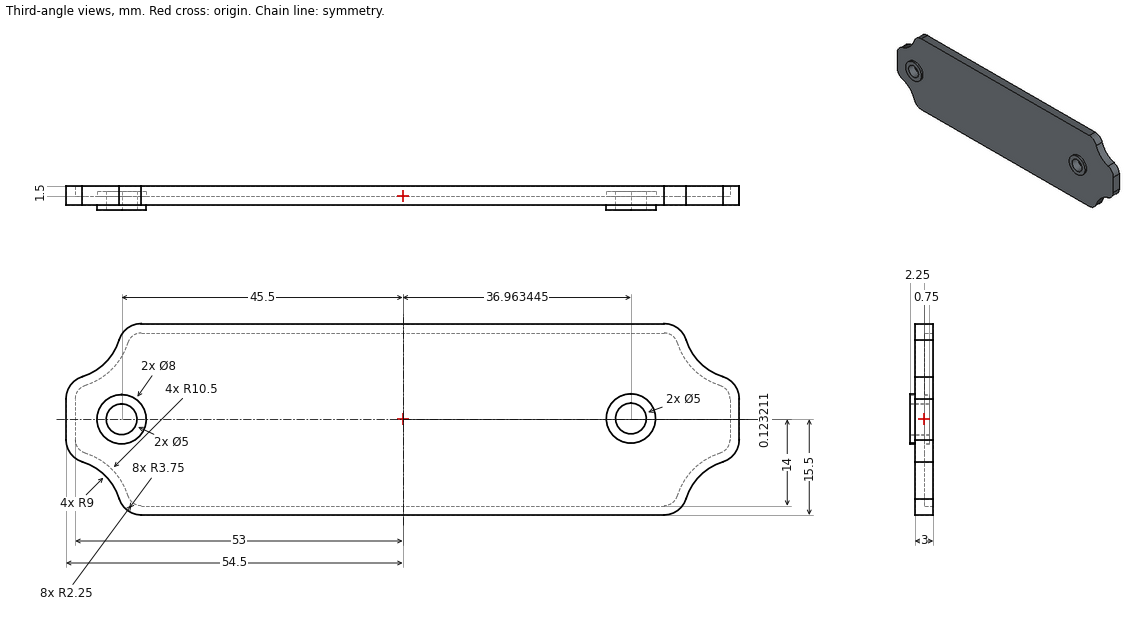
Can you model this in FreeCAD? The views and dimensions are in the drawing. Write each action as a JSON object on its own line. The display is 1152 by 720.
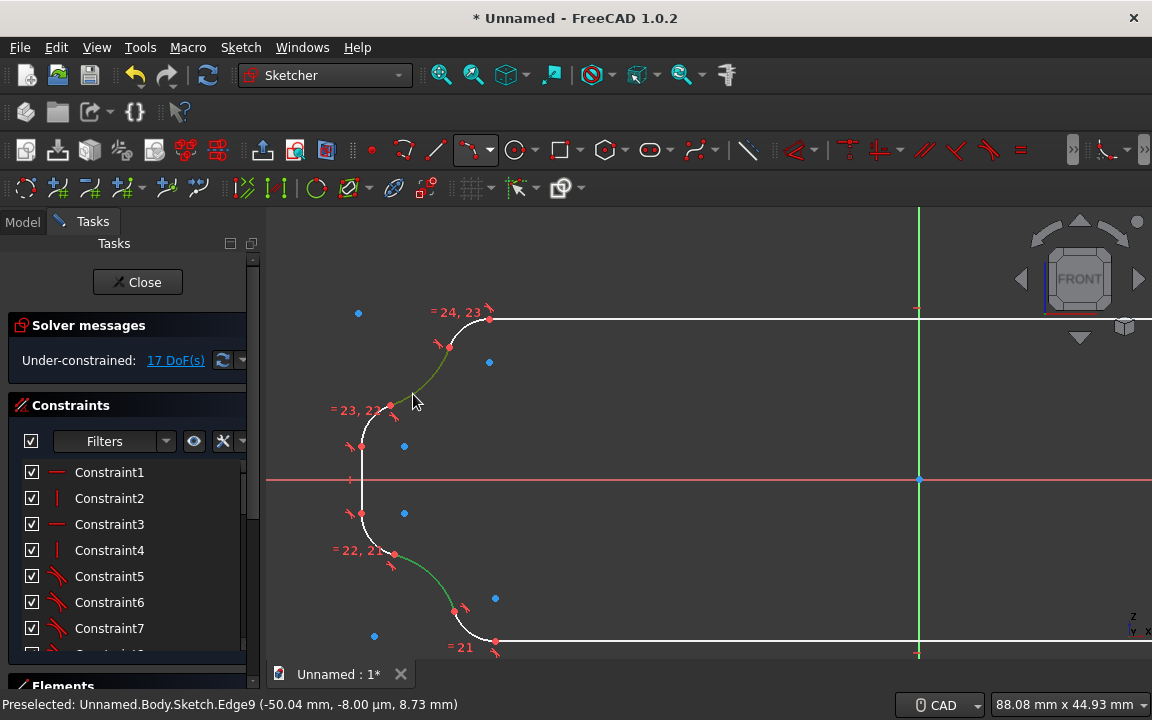
{"action": "scroll", "coordinate": [413, 395], "scroll_direction": "down", "scroll_amount": 4}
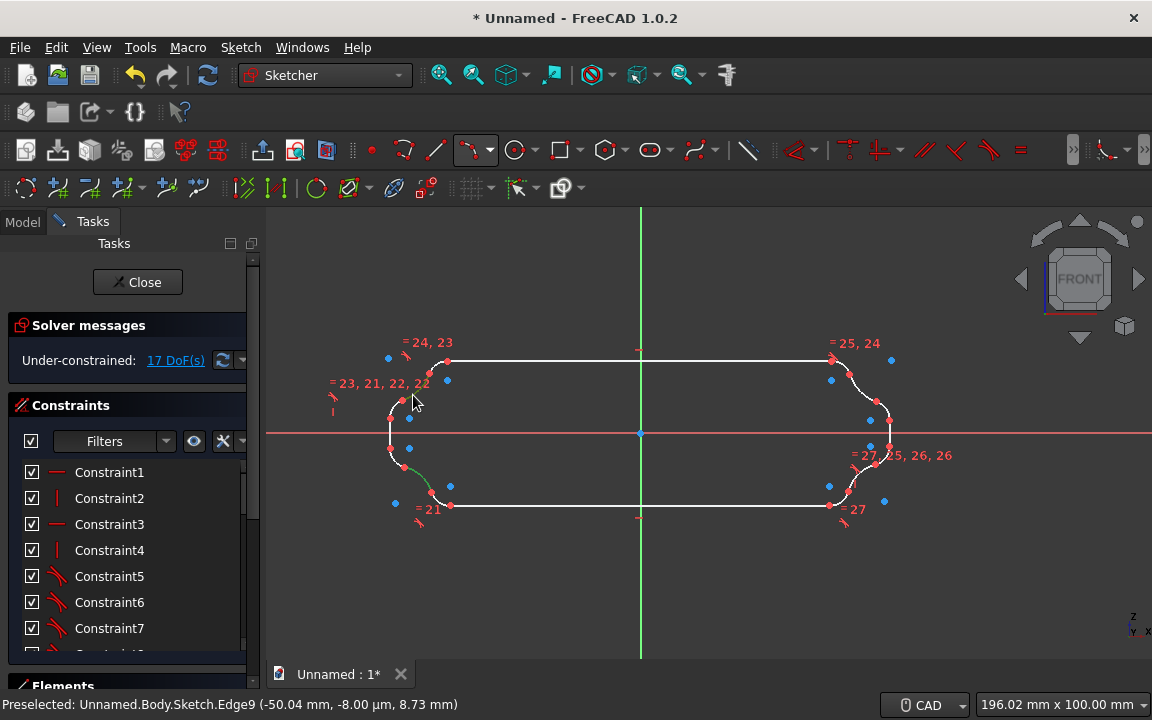
{"action": "left_click", "coordinate": [855, 385]}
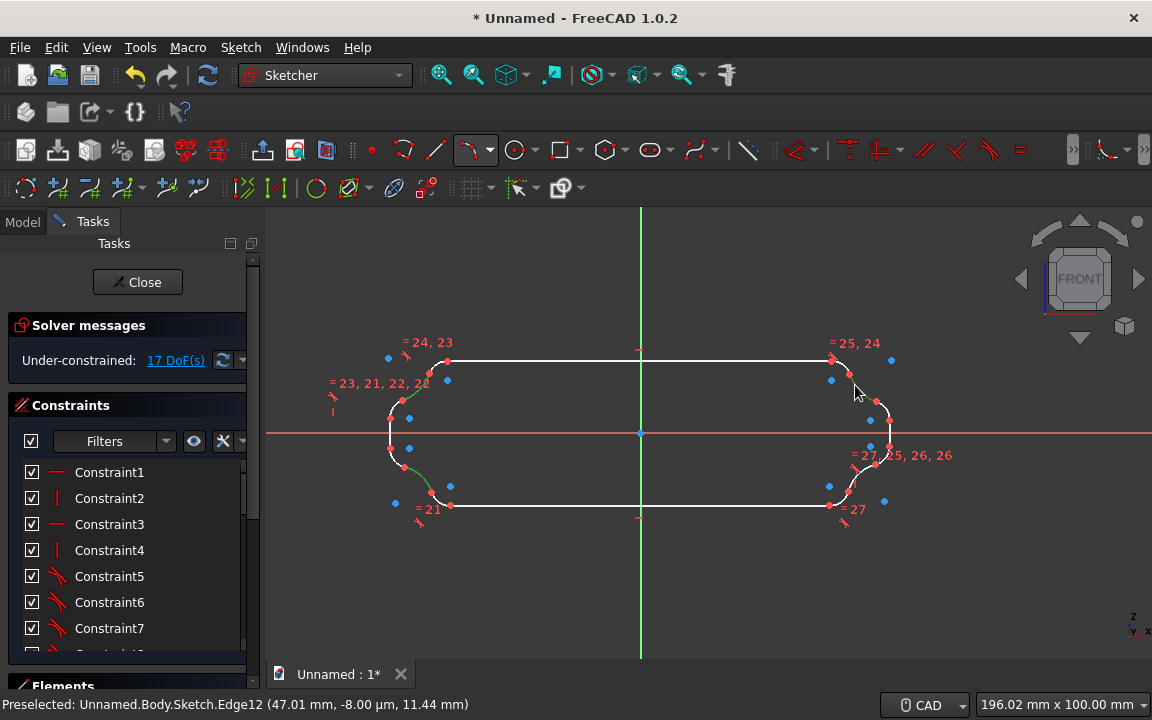
{"action": "scroll", "coordinate": [864, 470], "scroll_direction": "up", "scroll_amount": 4}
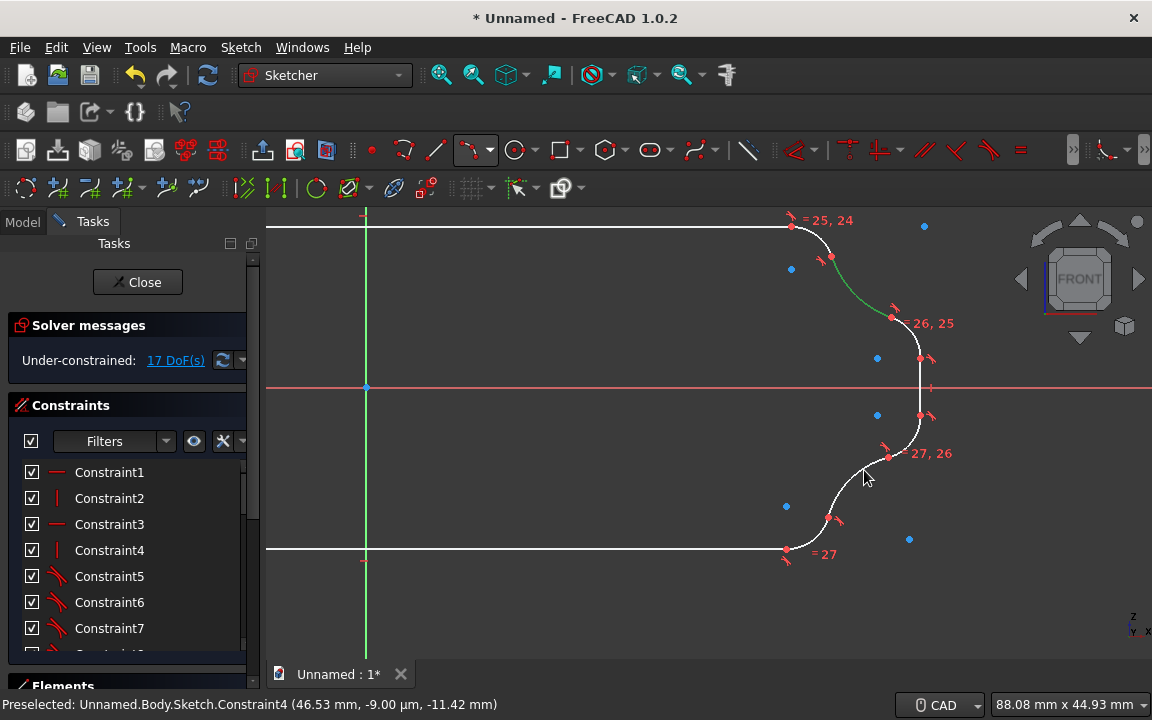
{"action": "left_click", "coordinate": [864, 468]}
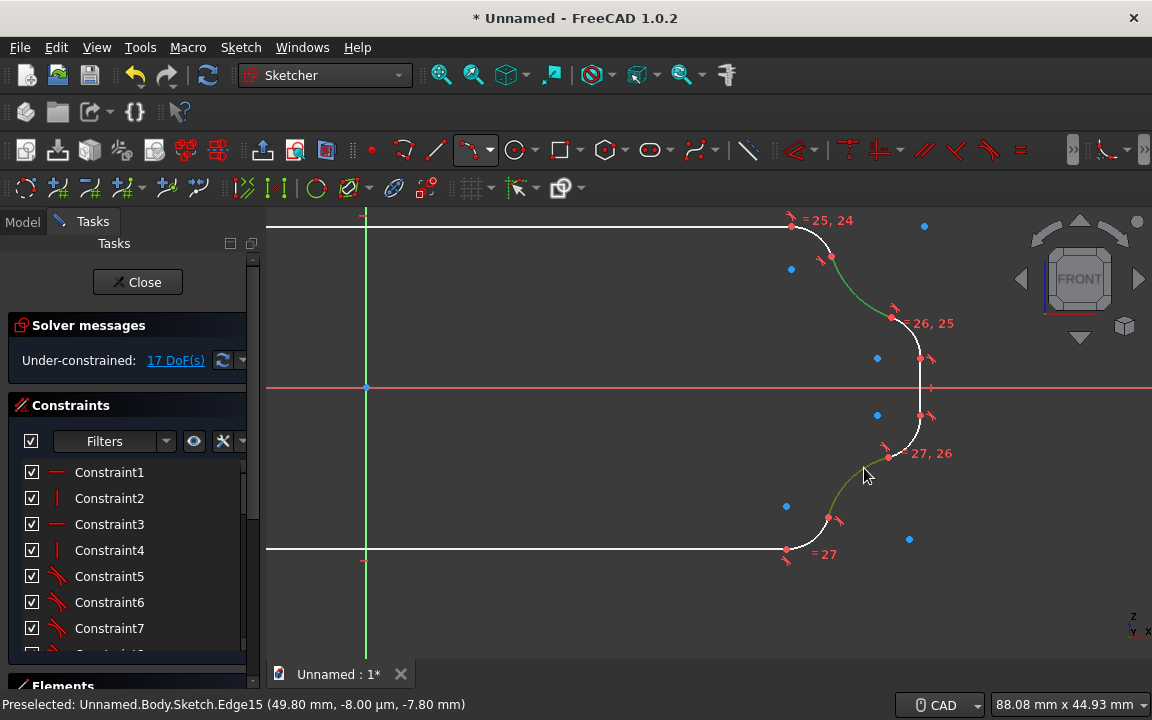
{"action": "left_click", "coordinate": [1022, 150]}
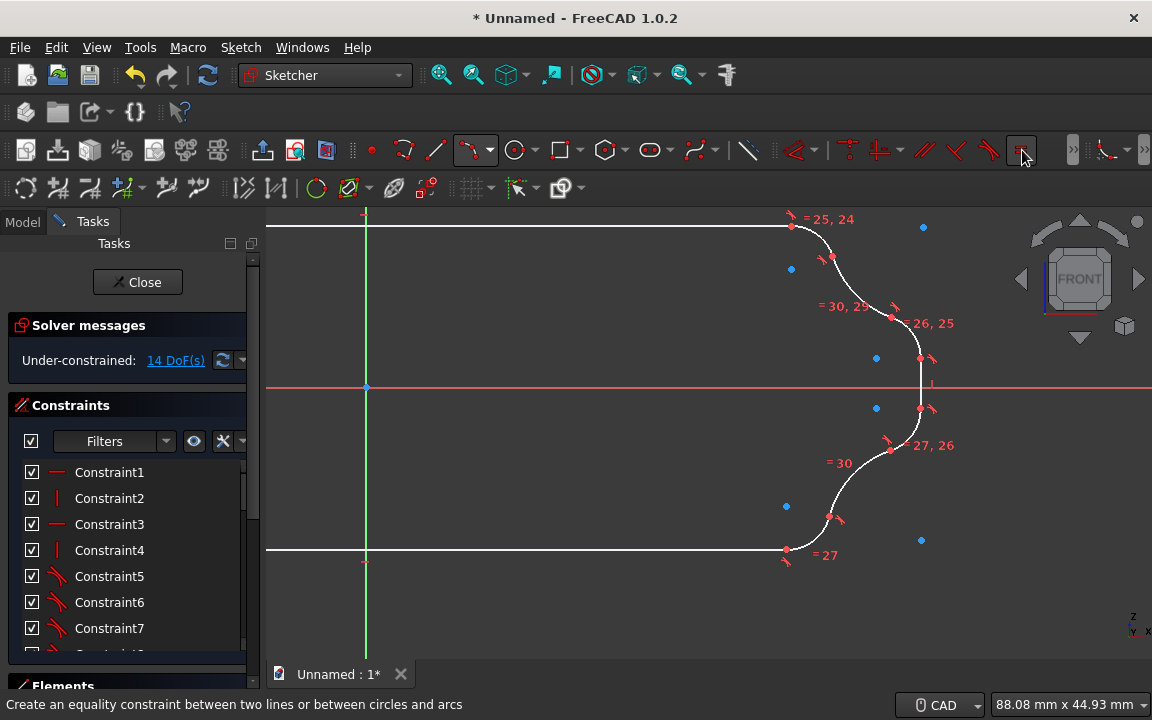
{"action": "scroll", "coordinate": [864, 470], "scroll_direction": "down", "scroll_amount": 4}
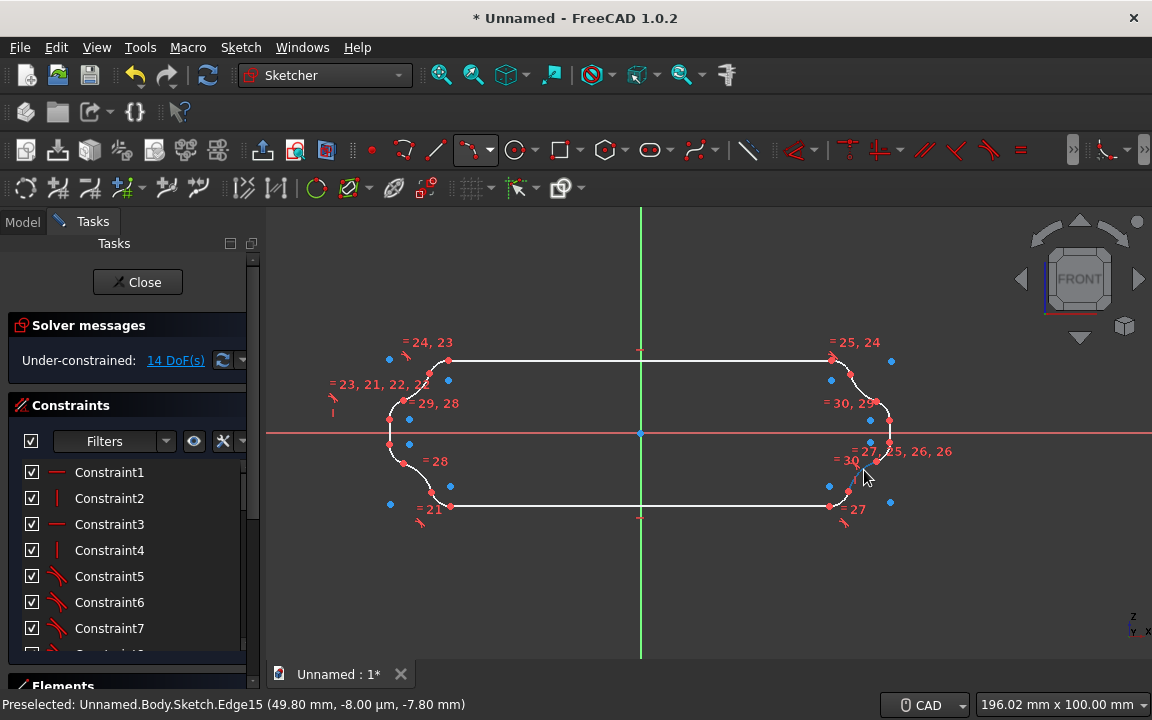
{"action": "left_click", "coordinate": [391, 505]}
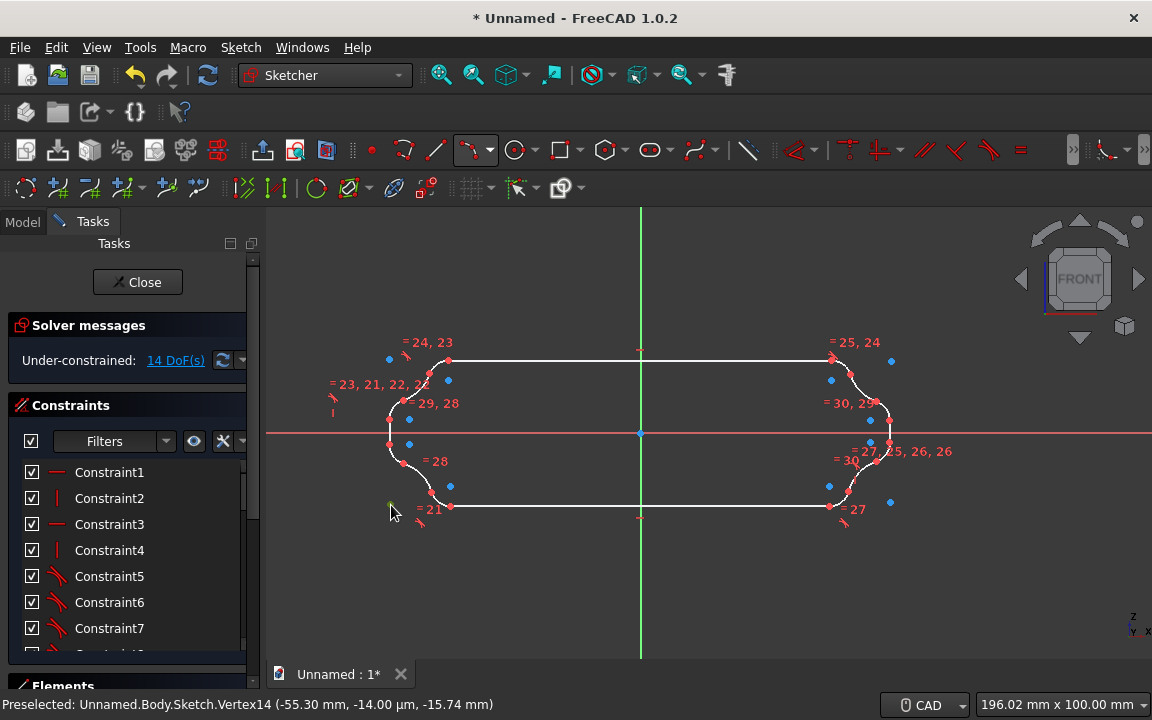
{"action": "left_click", "coordinate": [389, 360]}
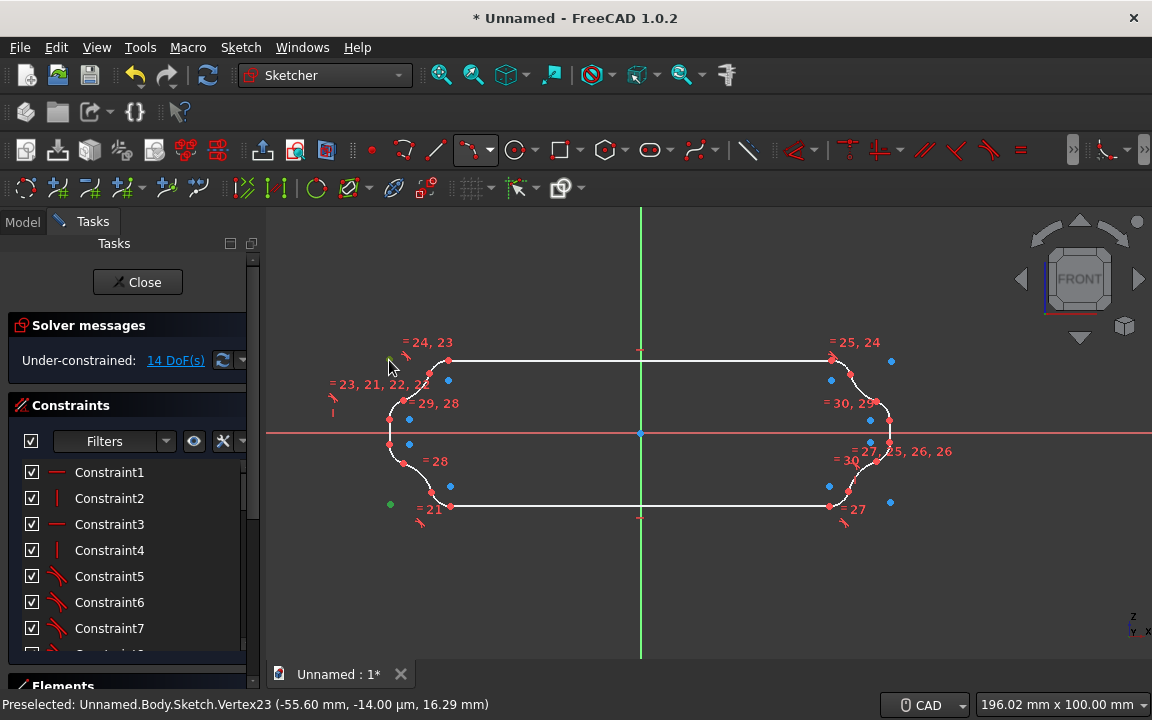
{"action": "left_click", "coordinate": [344, 433]}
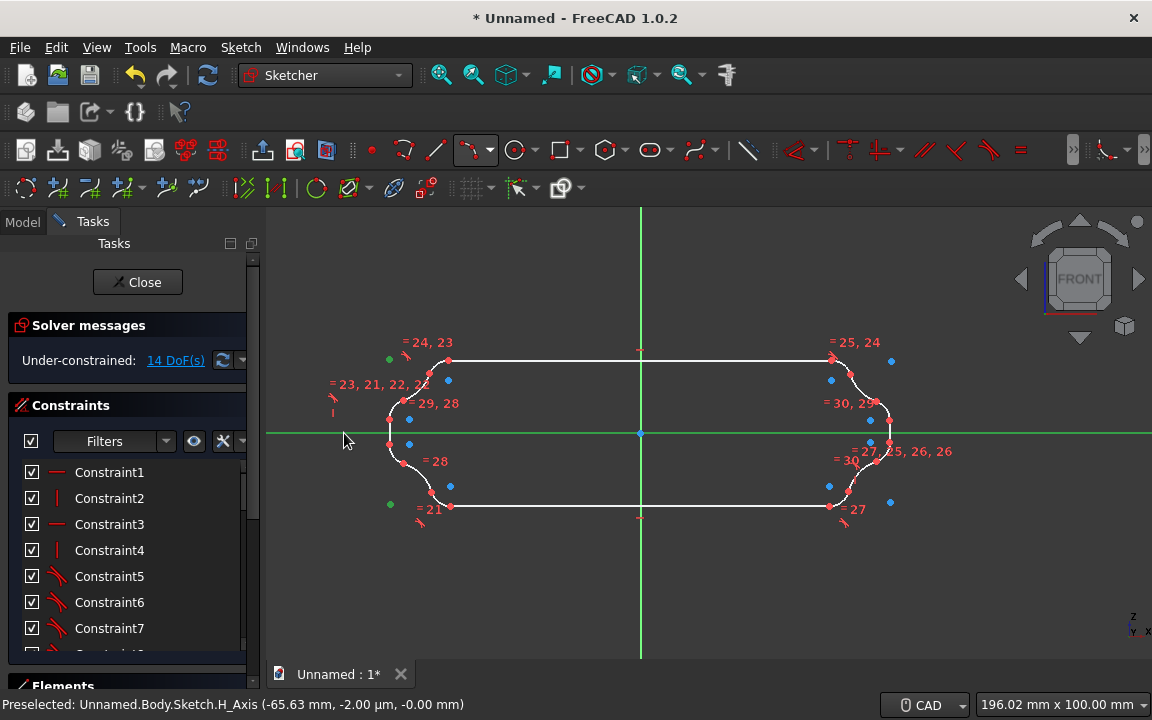
{"action": "key", "text": "s"}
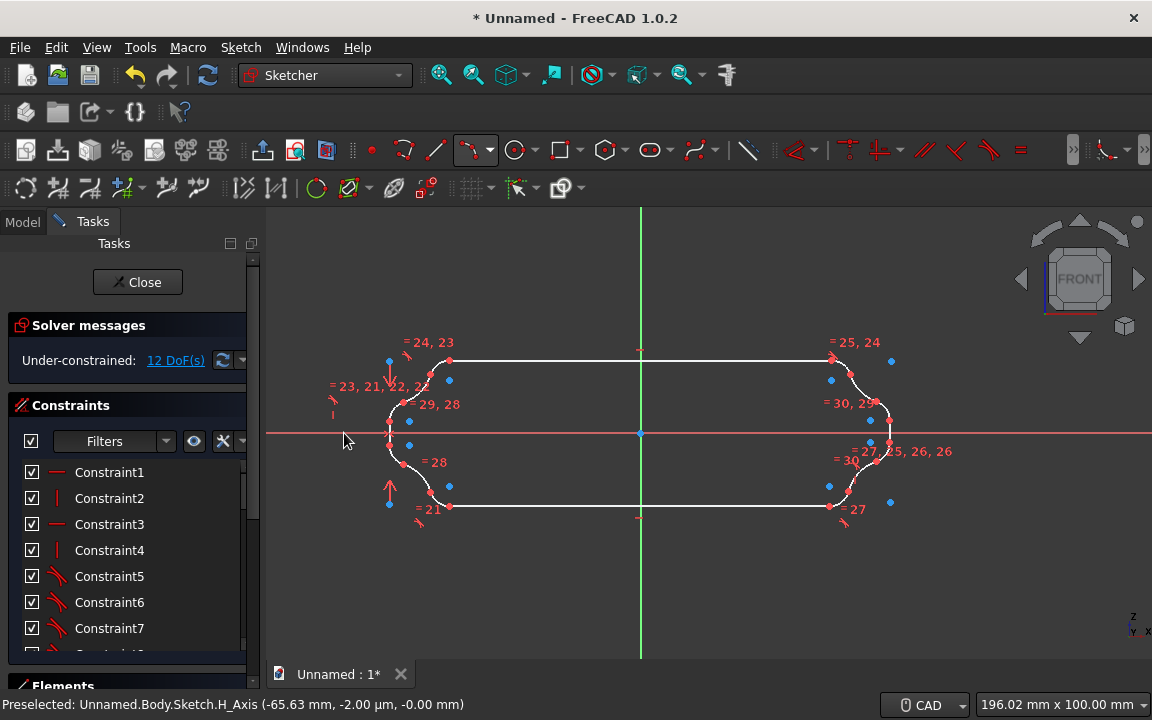
{"action": "left_click", "coordinate": [390, 362]}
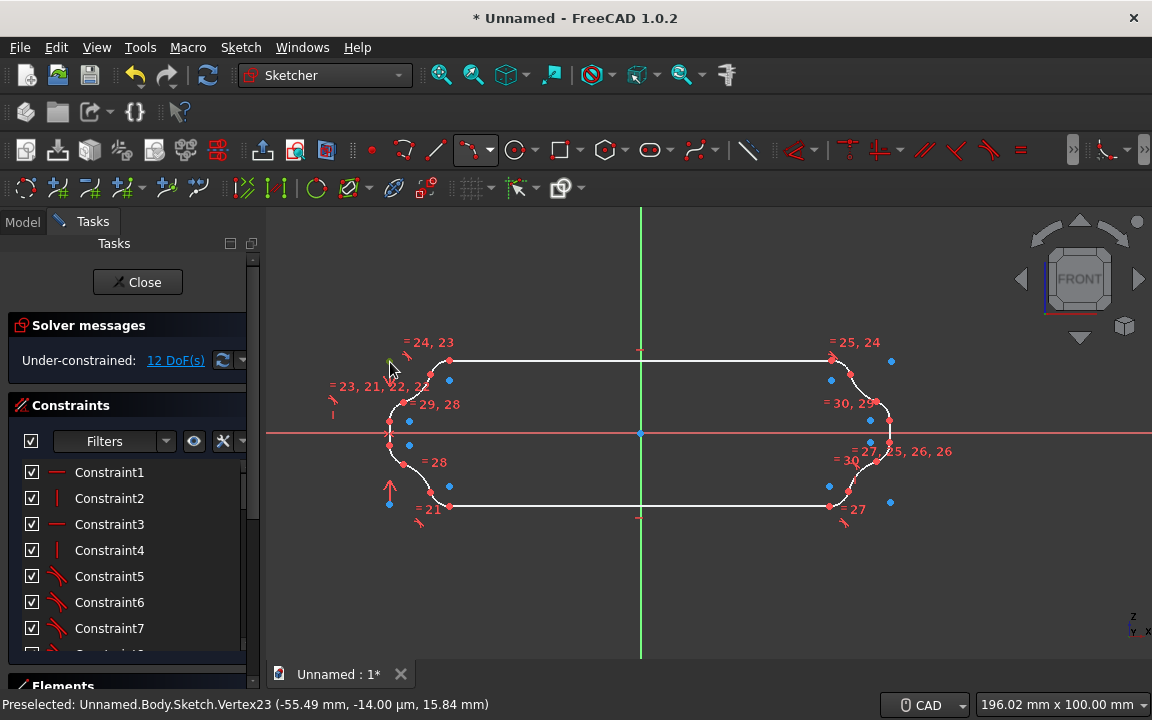
{"action": "left_click", "coordinate": [891, 361]}